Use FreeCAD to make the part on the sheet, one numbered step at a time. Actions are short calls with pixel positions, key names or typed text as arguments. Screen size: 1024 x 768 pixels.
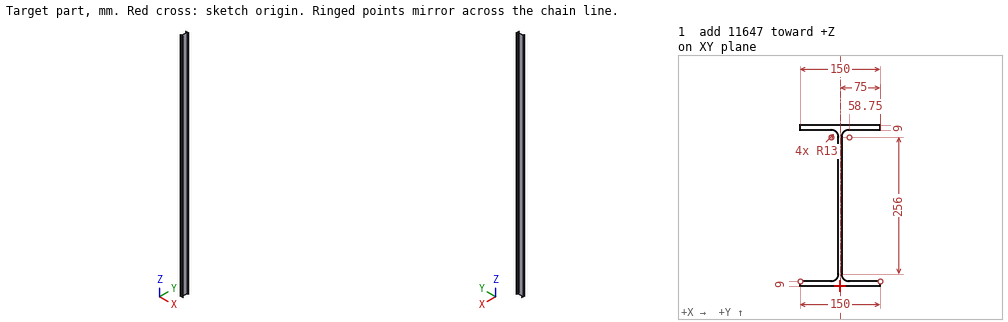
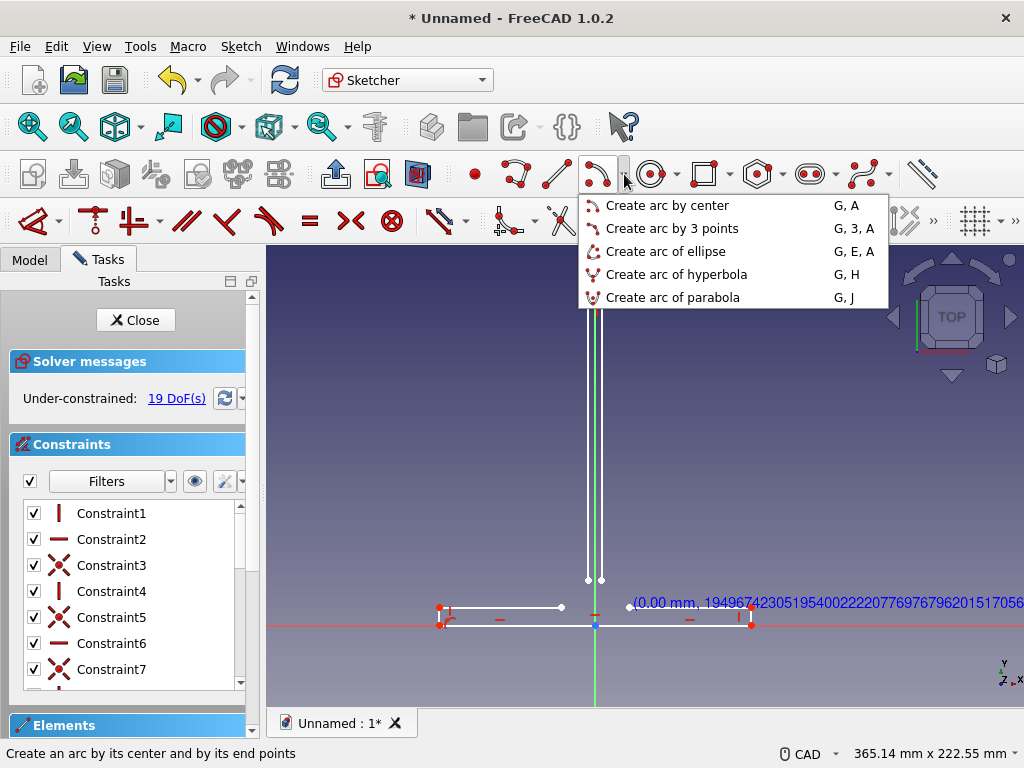
click(734, 228)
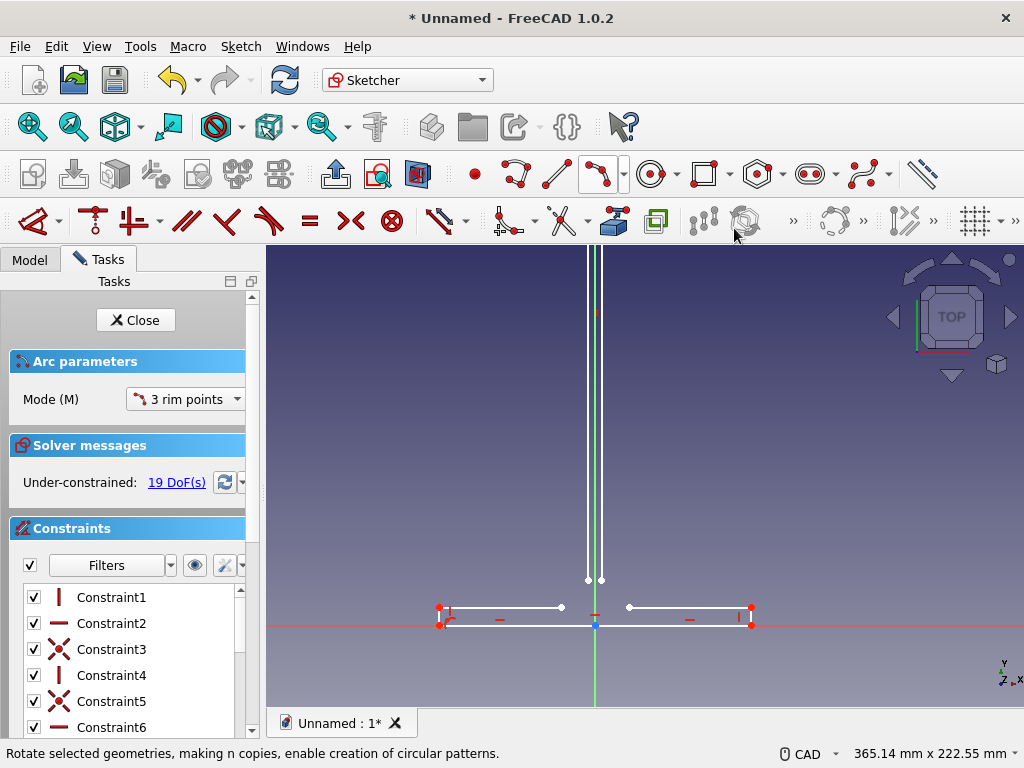
scroll(561, 608, down, 4)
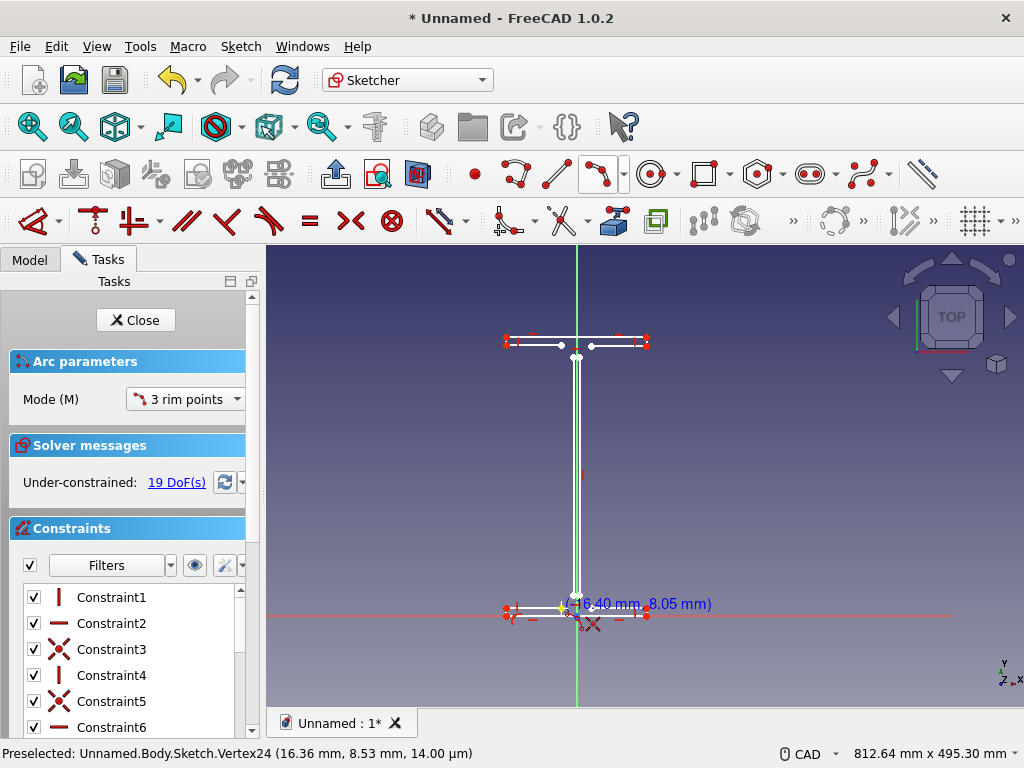
scroll(580, 357, up, 9)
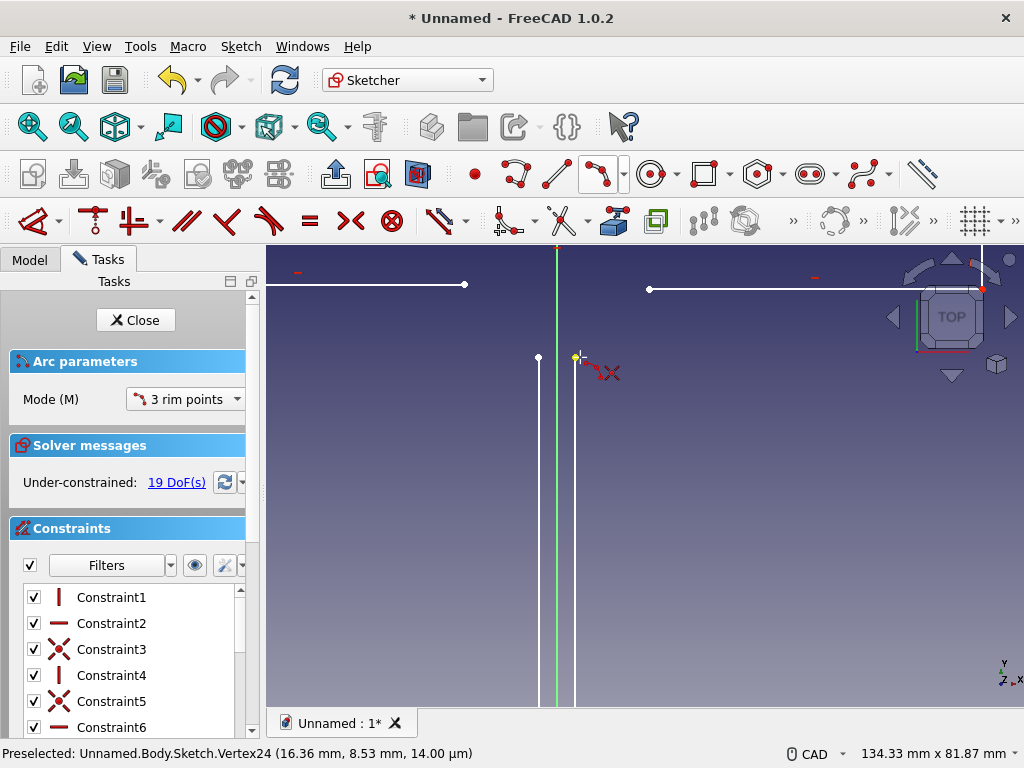
click(575, 357)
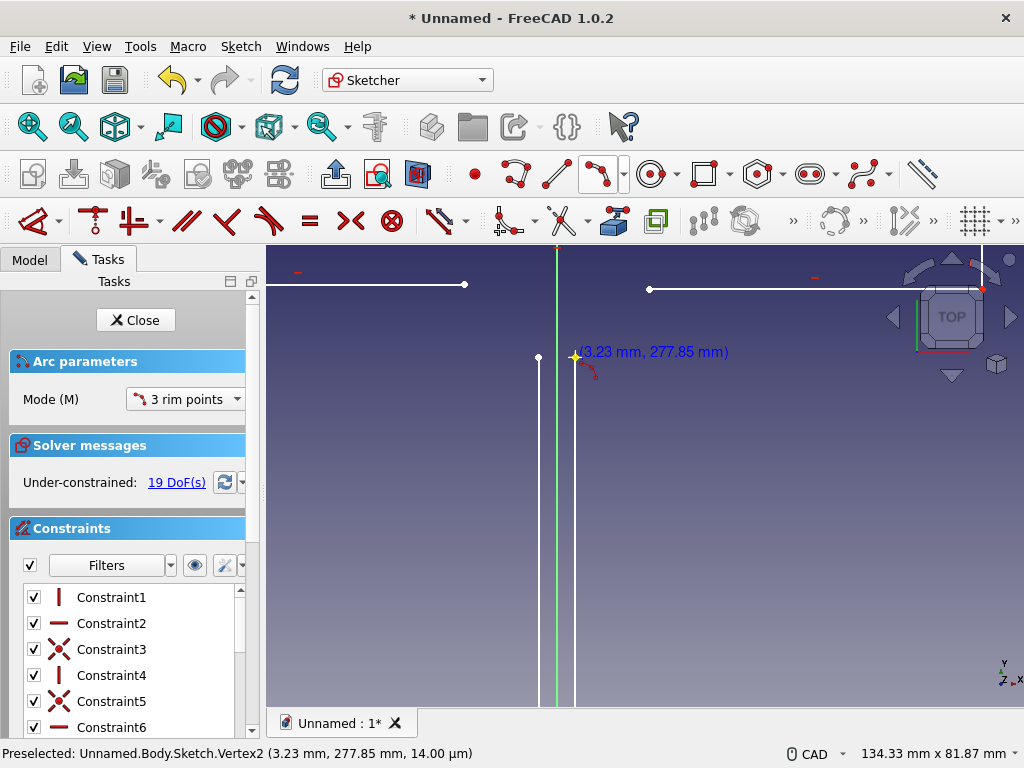
scroll(580, 357, down, 9)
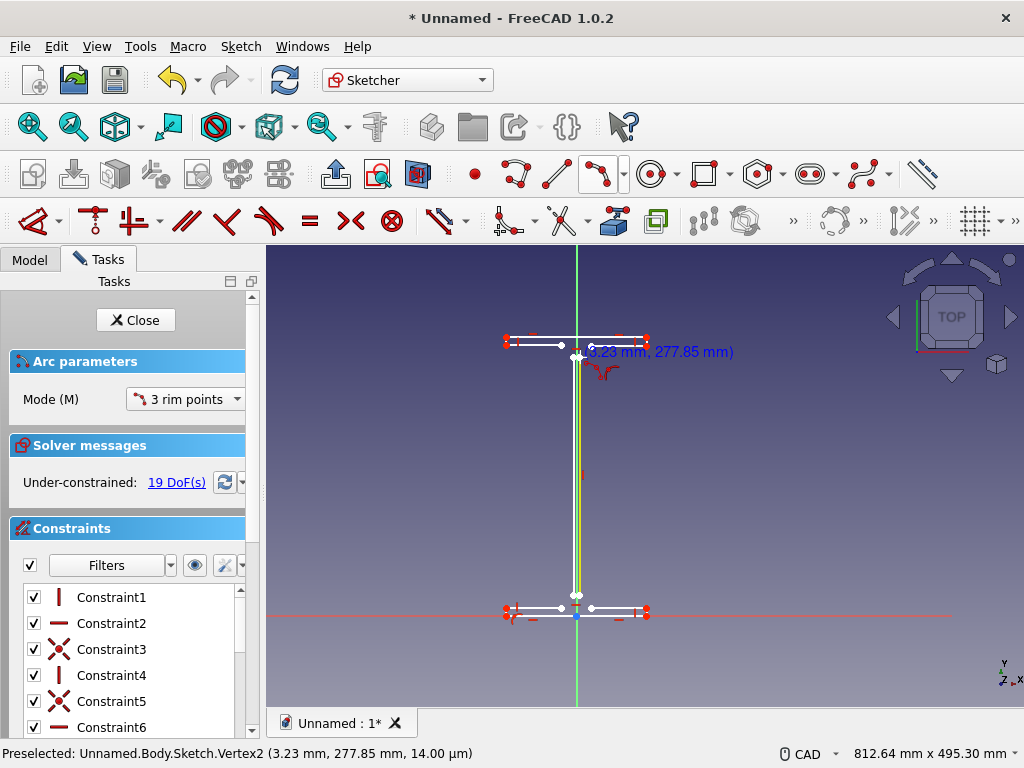
scroll(592, 345, up, 4)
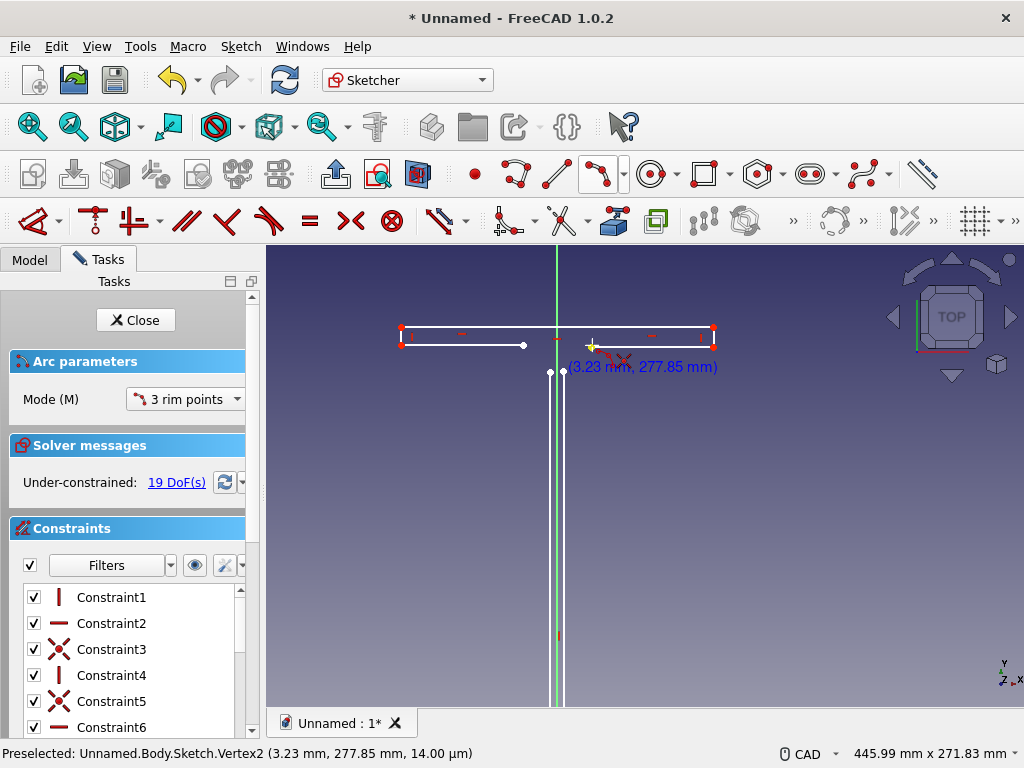
click(591, 347)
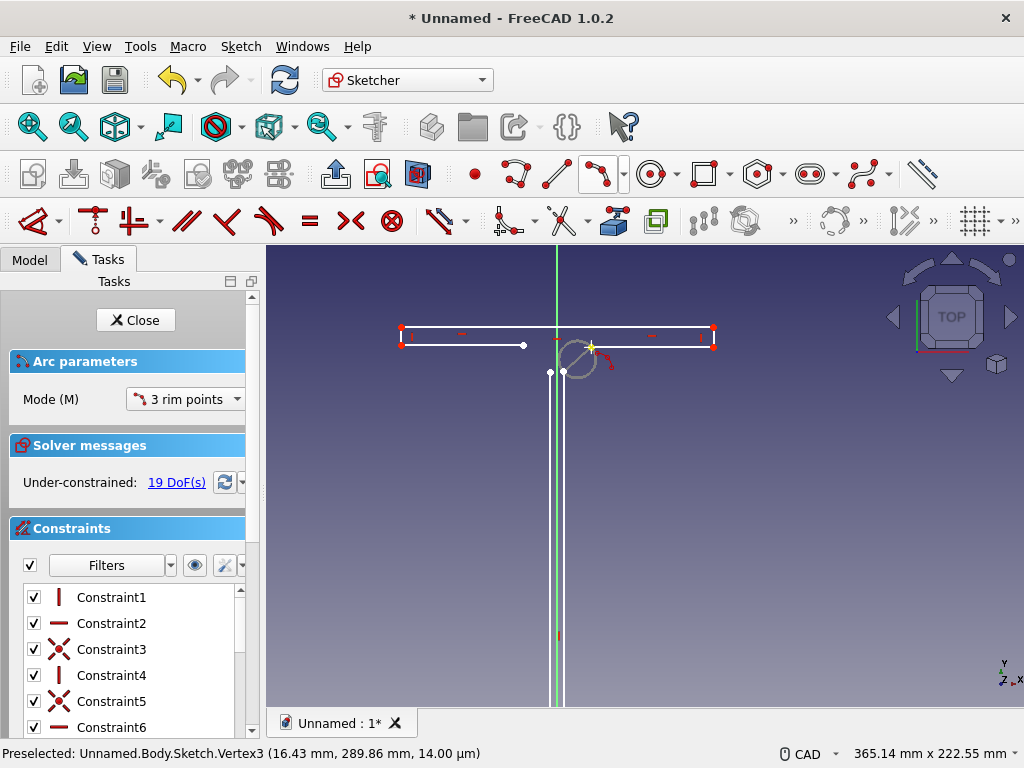
scroll(572, 353, up, 4)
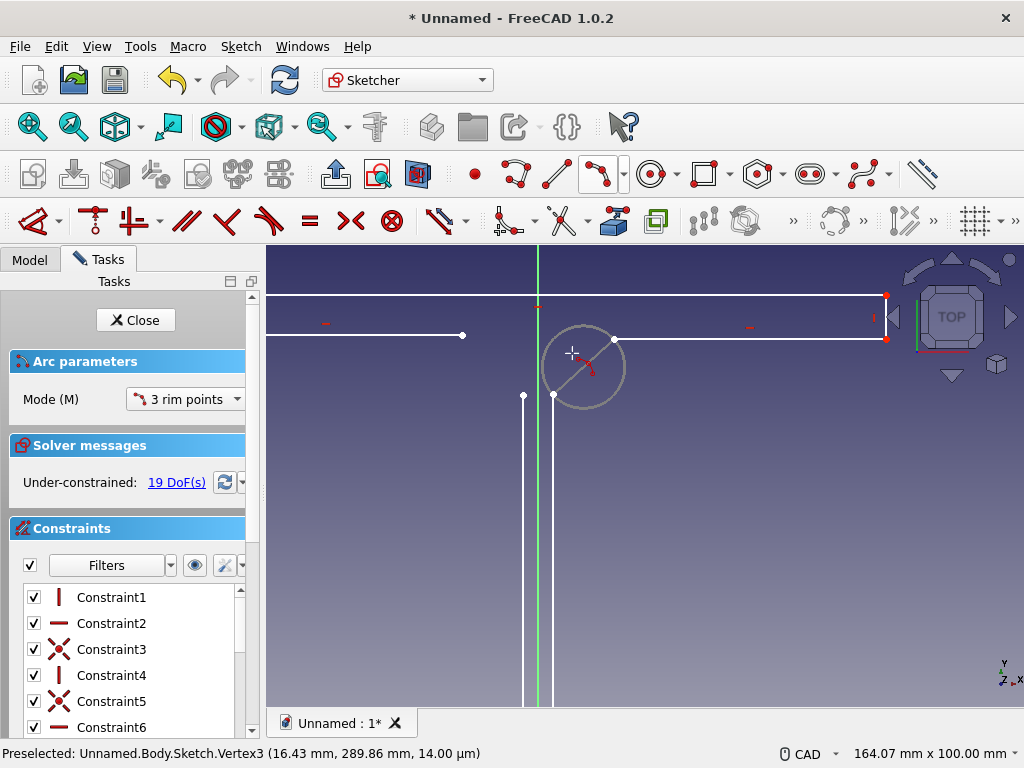
click(571, 352)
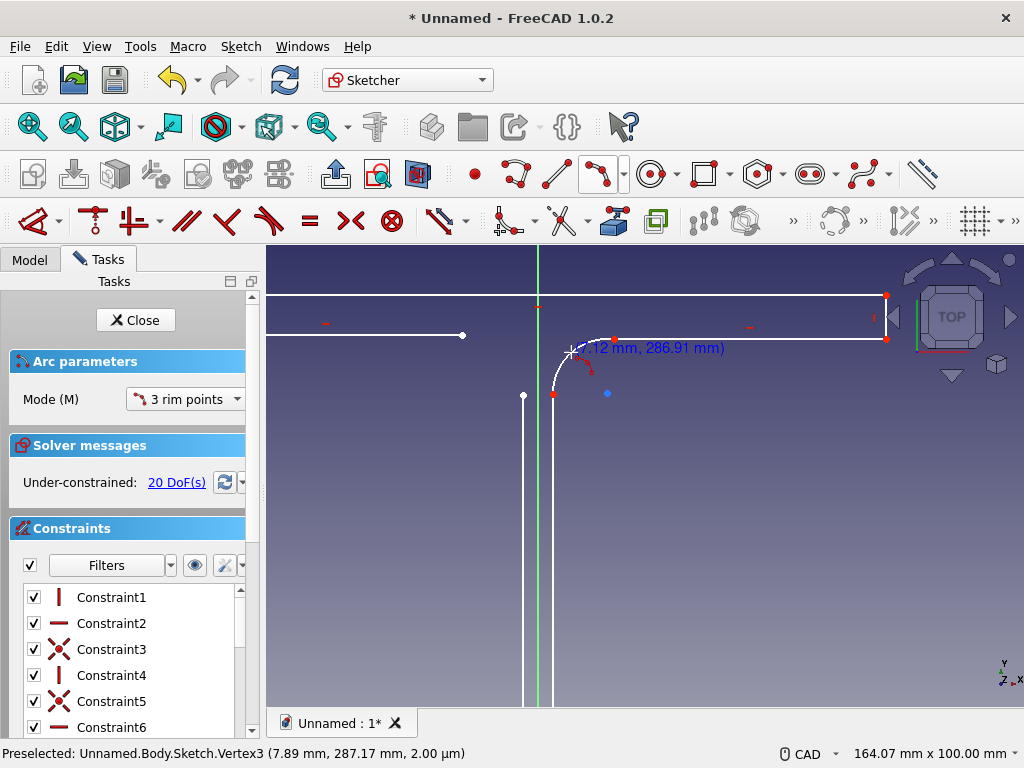
click(463, 335)
click(523, 395)
click(506, 352)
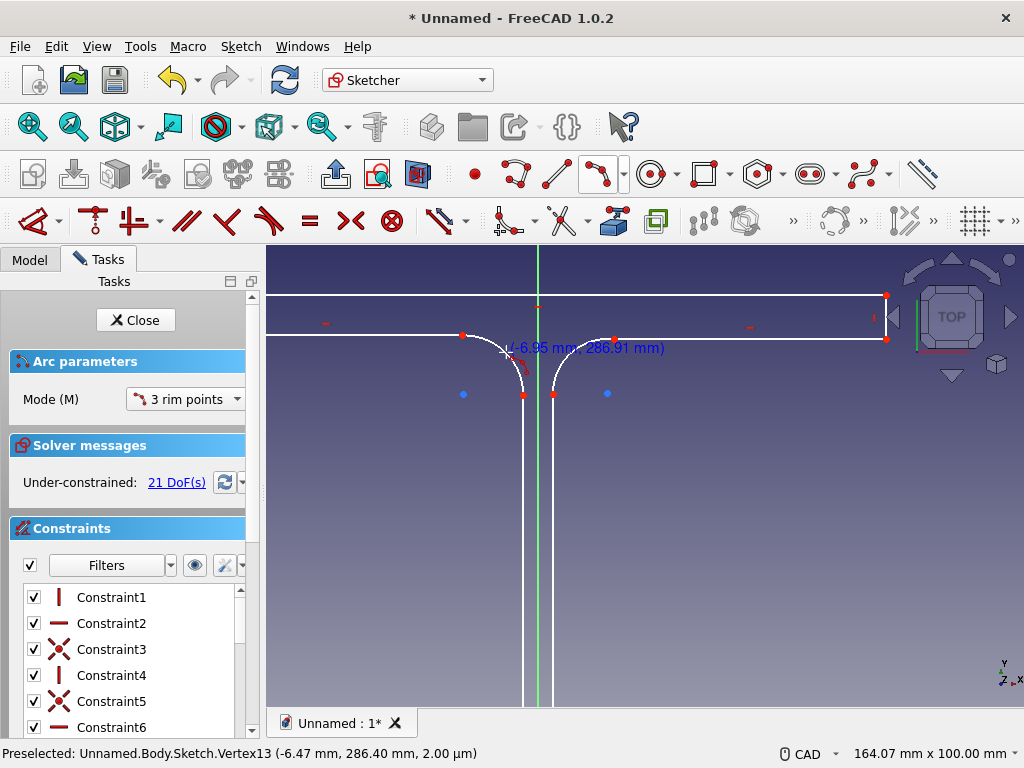
scroll(586, 347, down, 8)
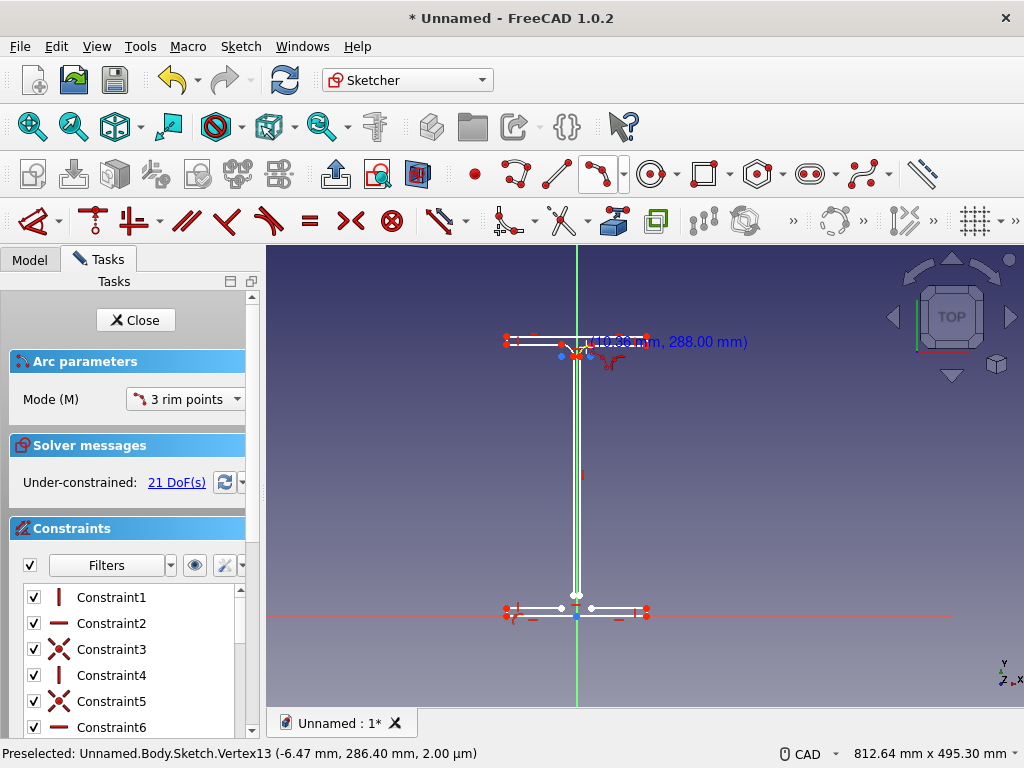
scroll(574, 595, up, 9)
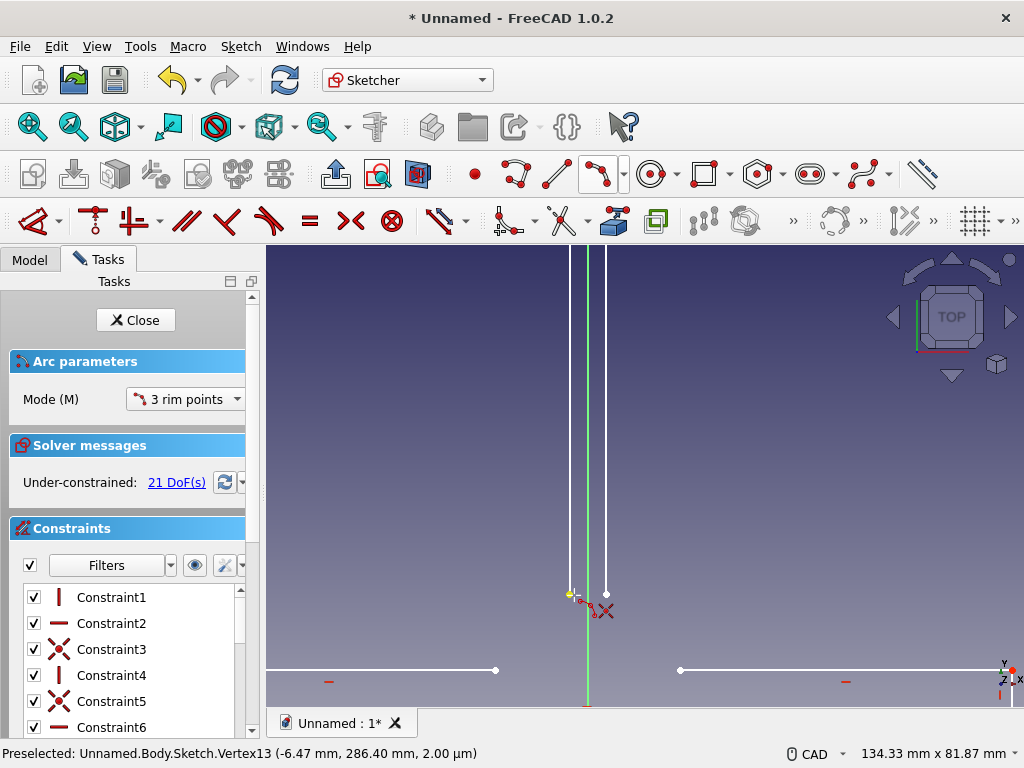
click(570, 595)